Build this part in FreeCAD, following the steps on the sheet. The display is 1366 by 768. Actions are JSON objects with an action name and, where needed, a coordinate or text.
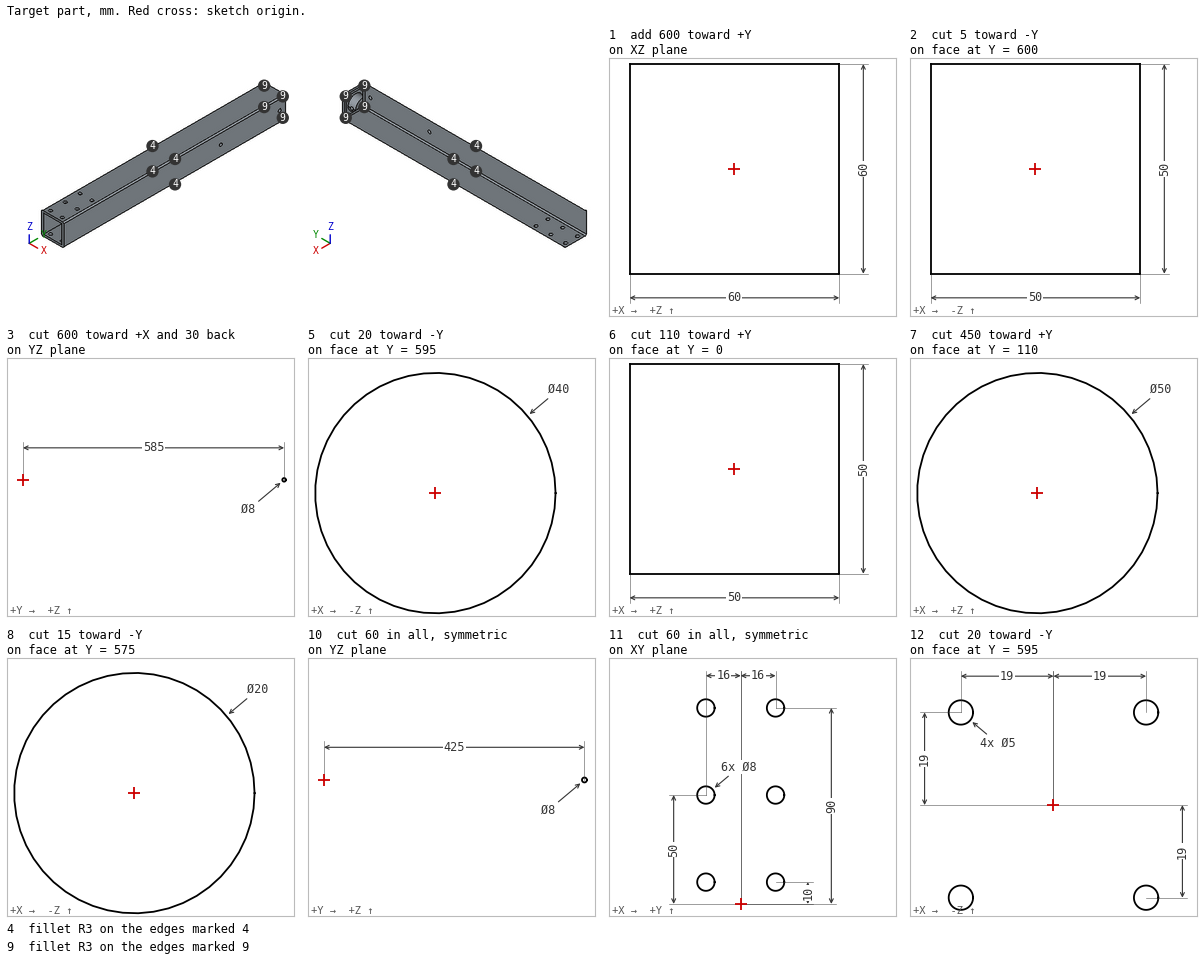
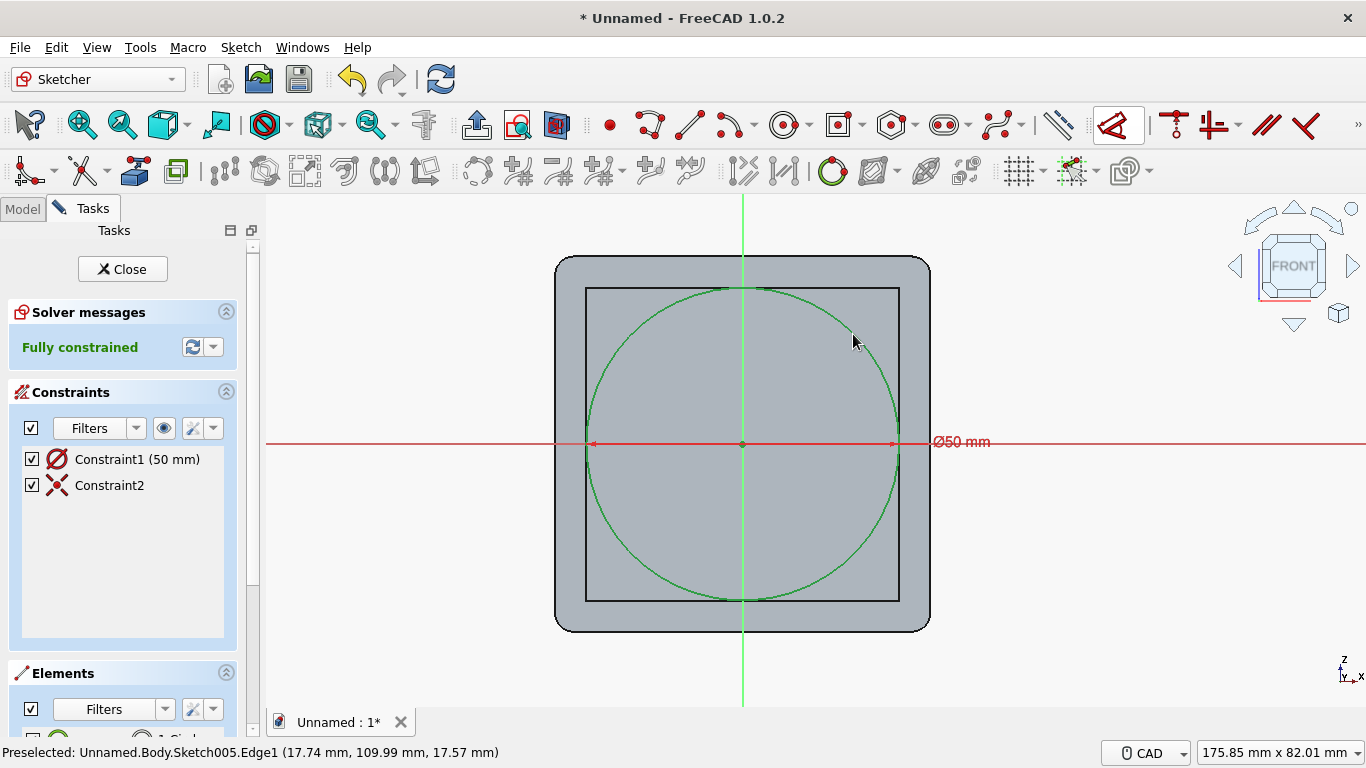
{"action": "left_click", "coordinate": [123, 269]}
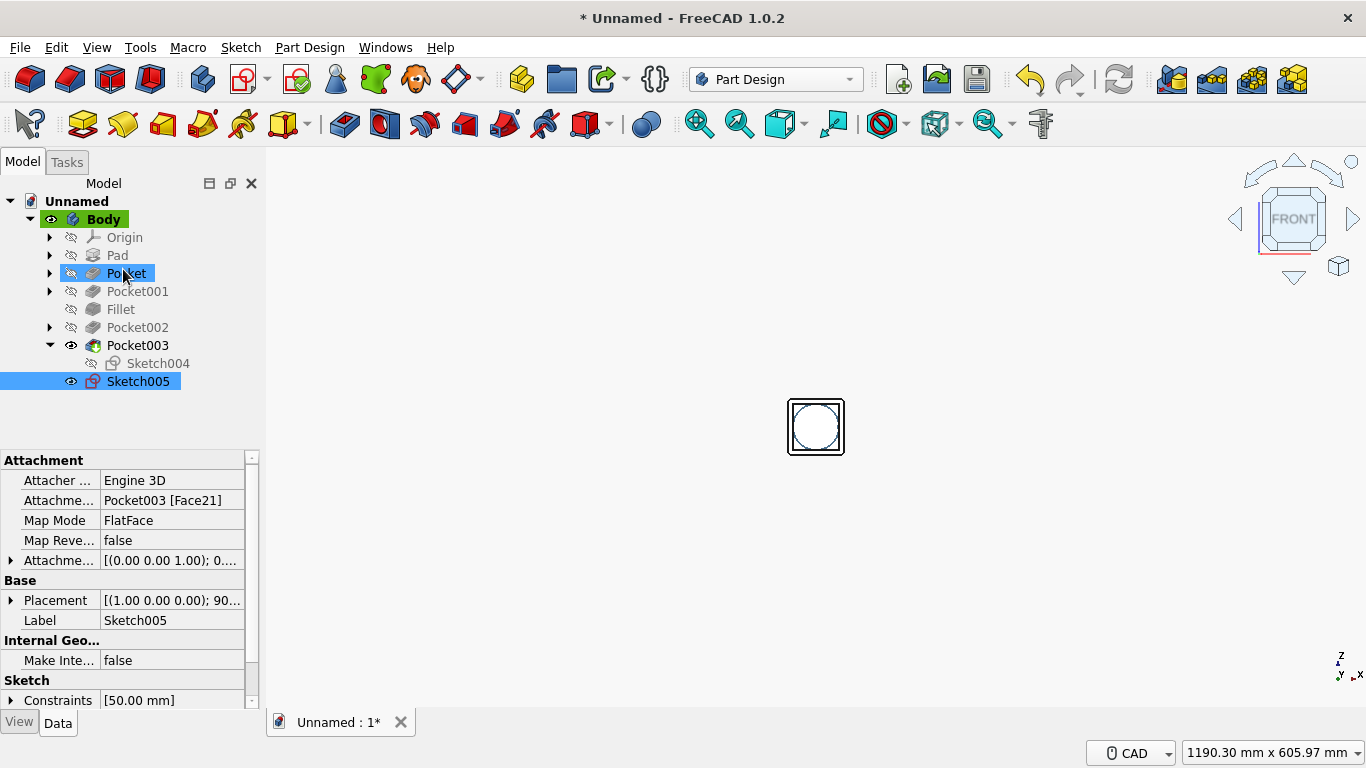
{"action": "left_click", "coordinate": [346, 124]}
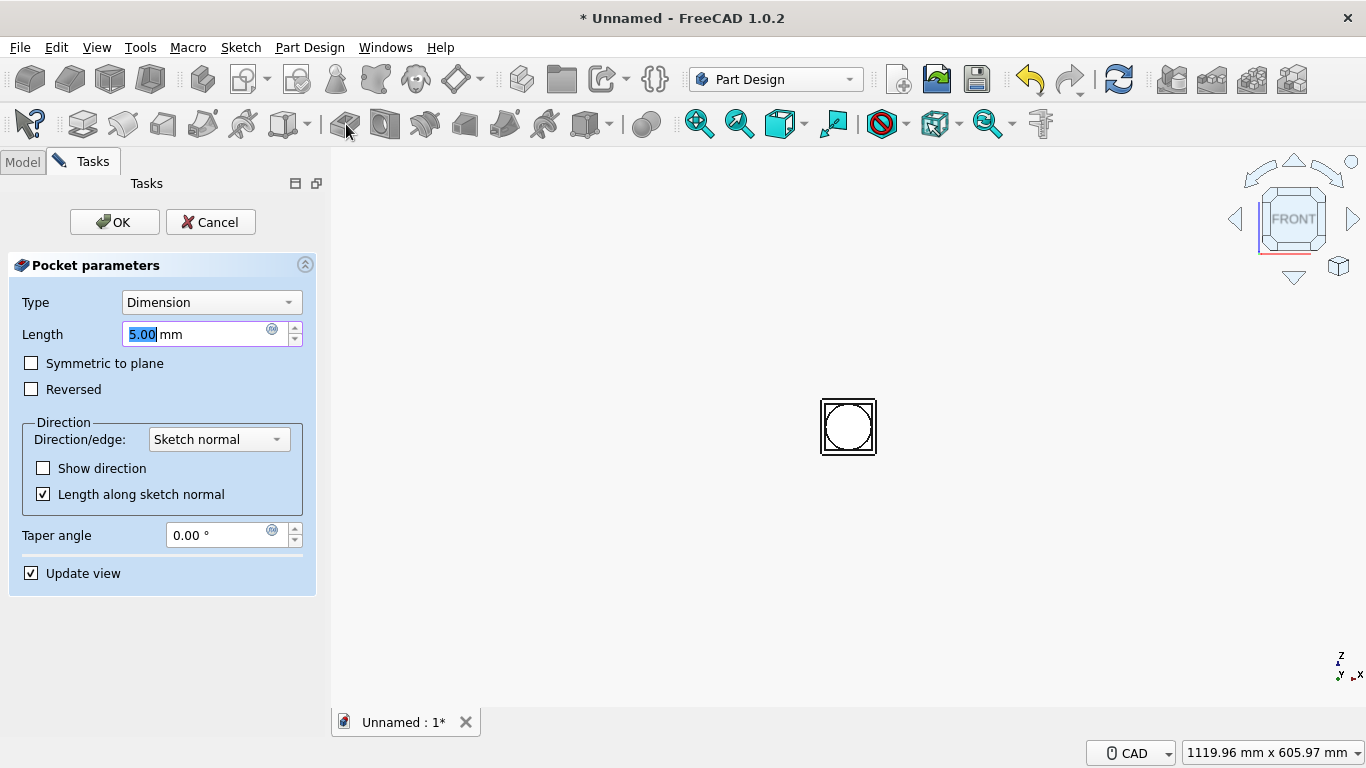
{"action": "type", "text": "450"}
{"action": "key", "text": "Tab"}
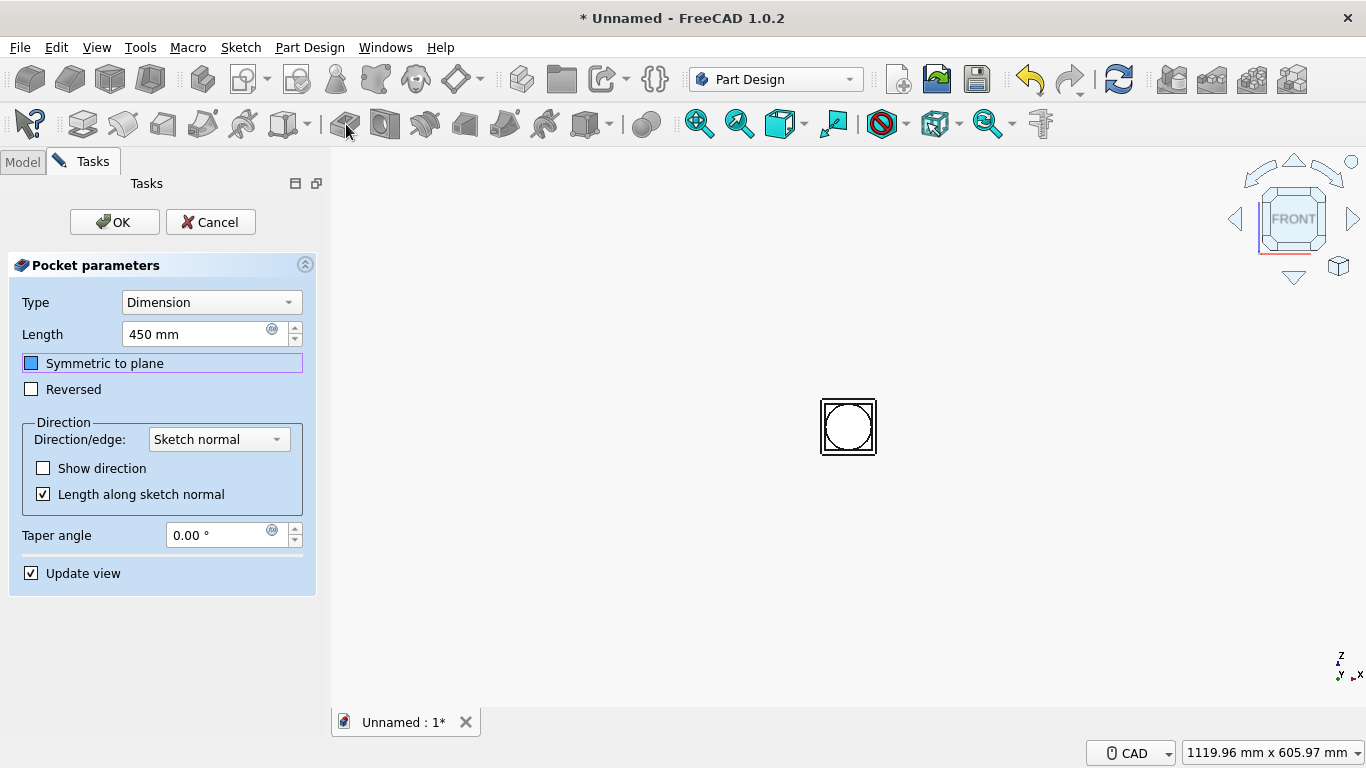
{"action": "left_click", "coordinate": [115, 222]}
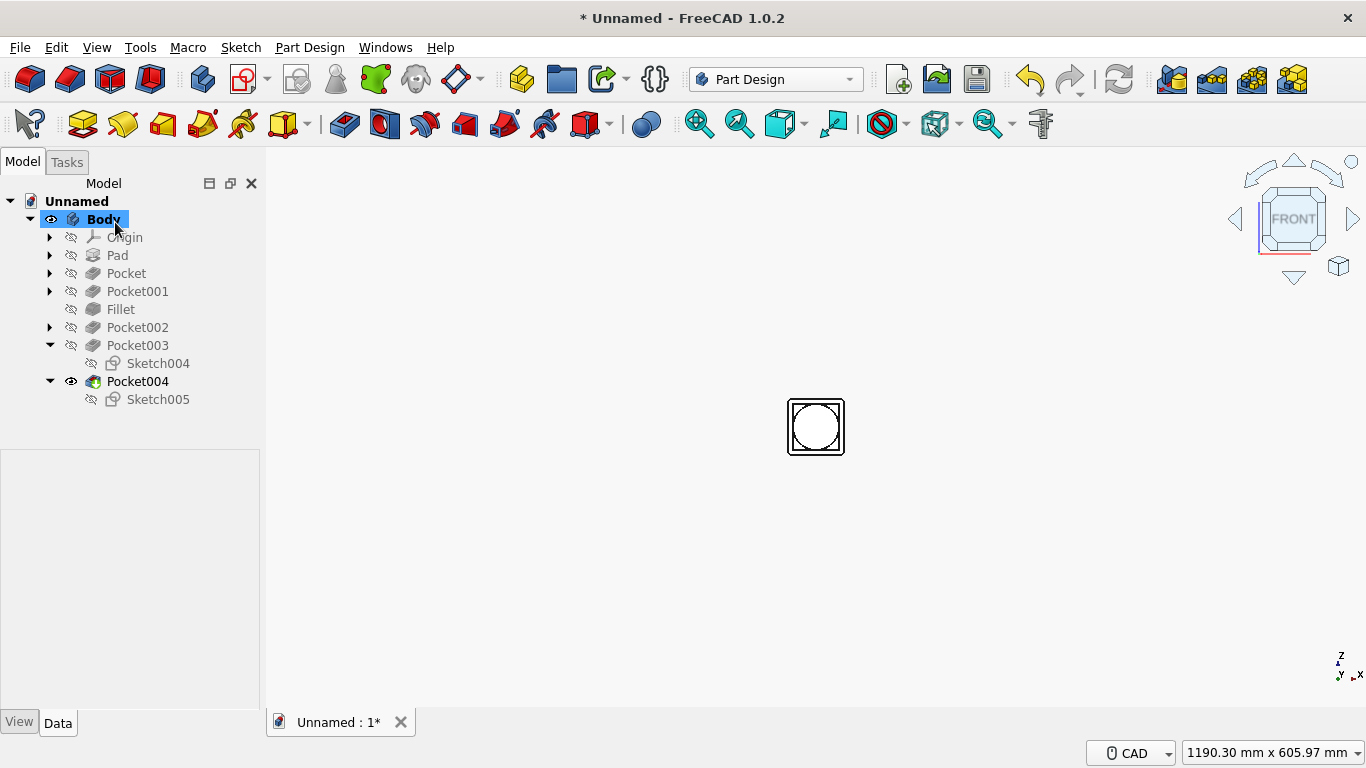
{"action": "key", "text": "v f"}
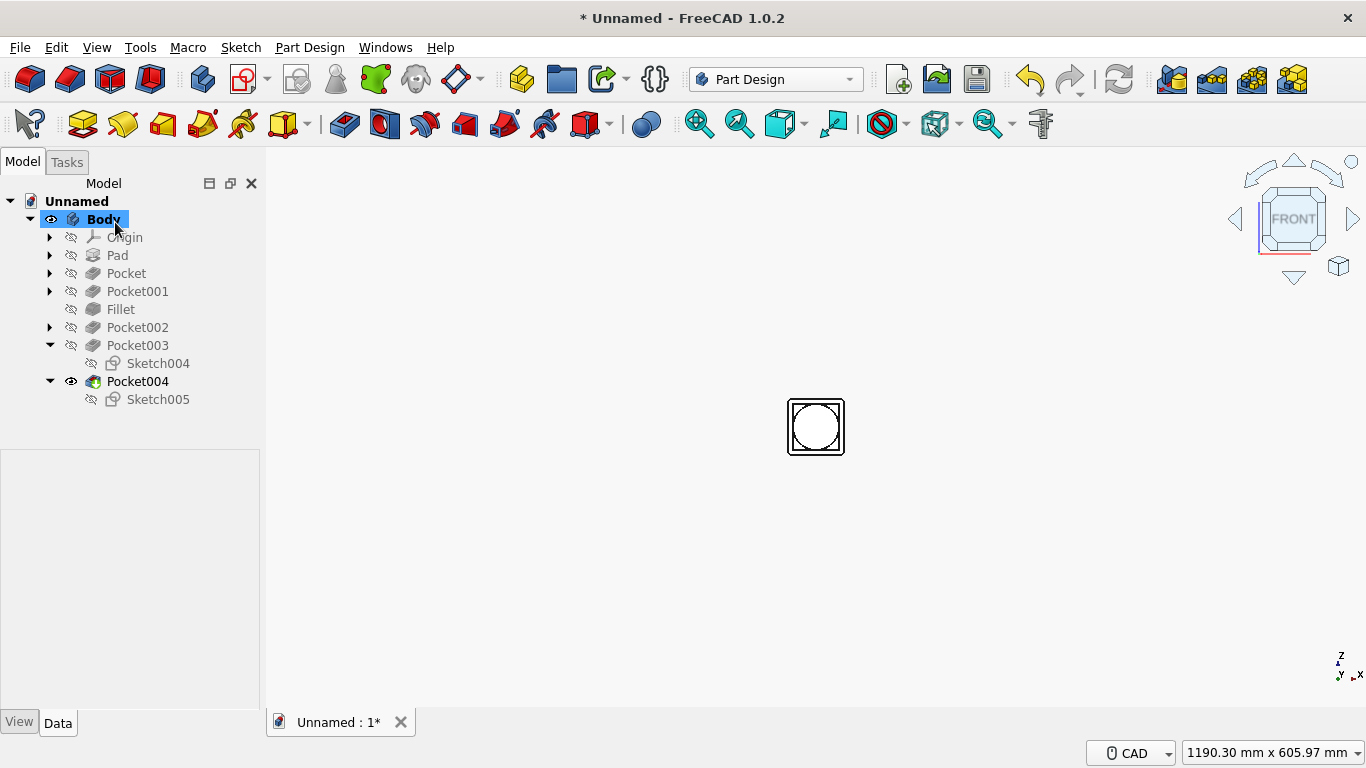
{"action": "key", "text": "4"}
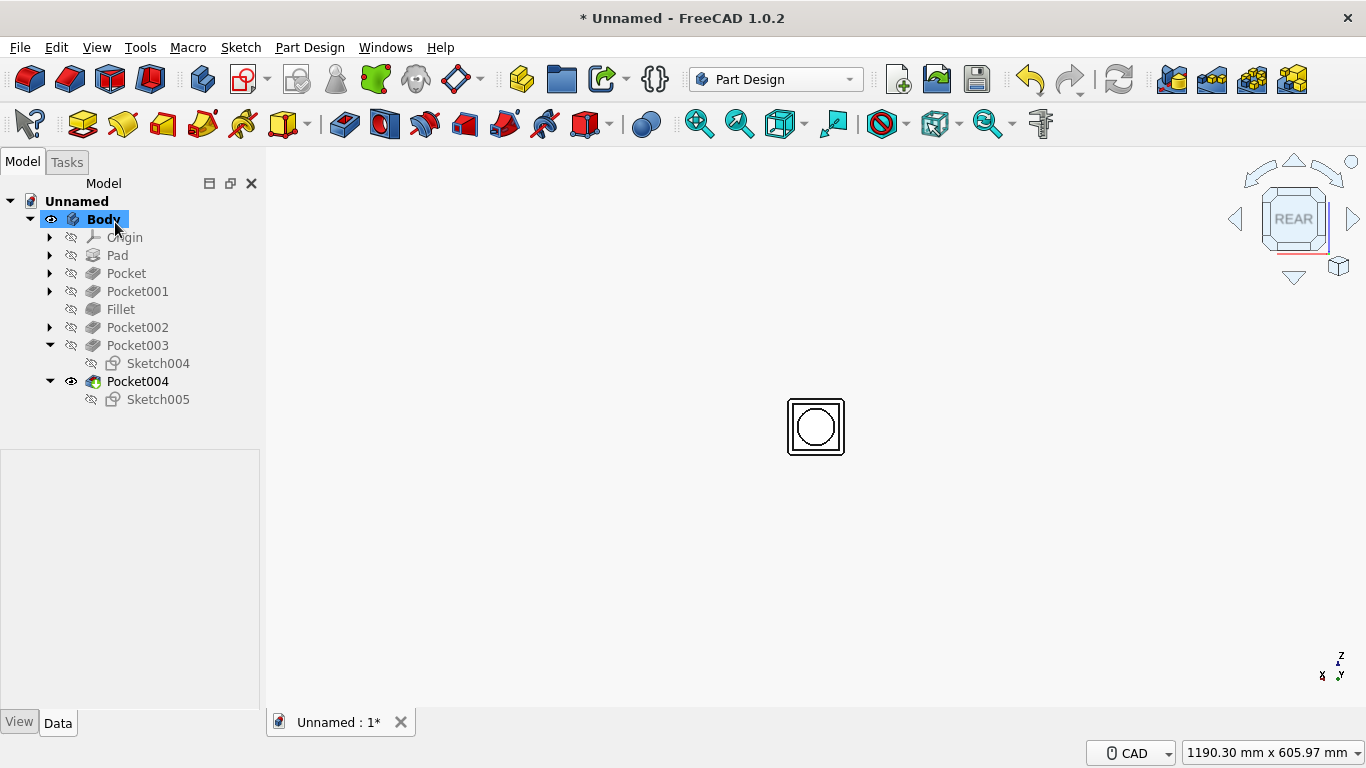
{"action": "left_click", "coordinate": [700, 124]}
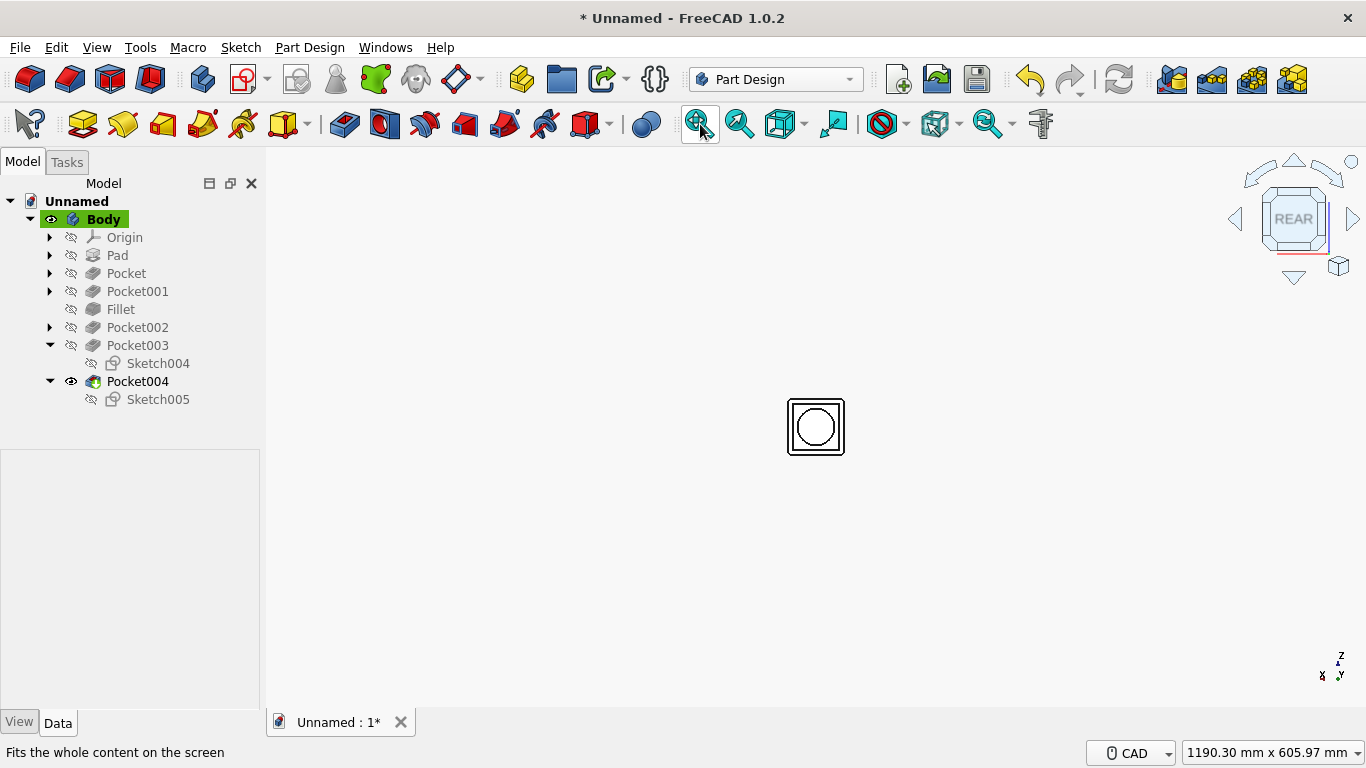
{"action": "left_click", "coordinate": [816, 426]}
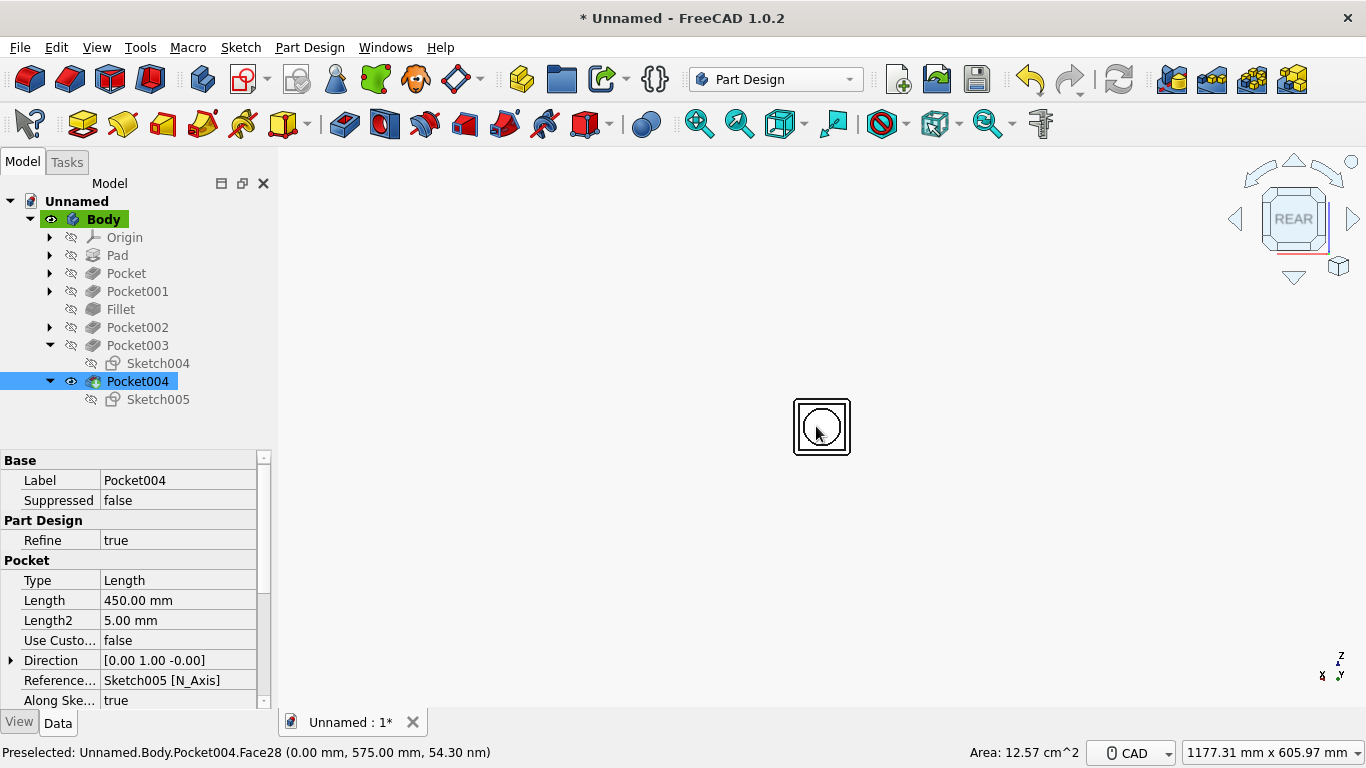
{"action": "left_click", "coordinate": [244, 80]}